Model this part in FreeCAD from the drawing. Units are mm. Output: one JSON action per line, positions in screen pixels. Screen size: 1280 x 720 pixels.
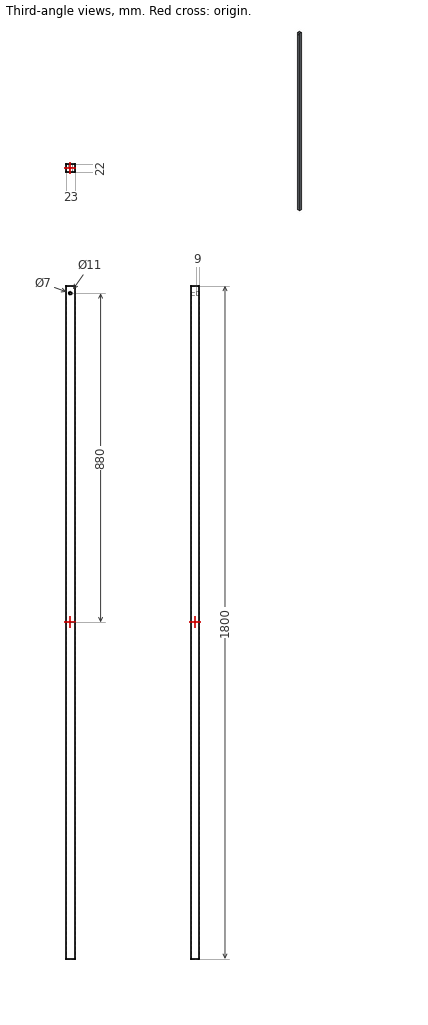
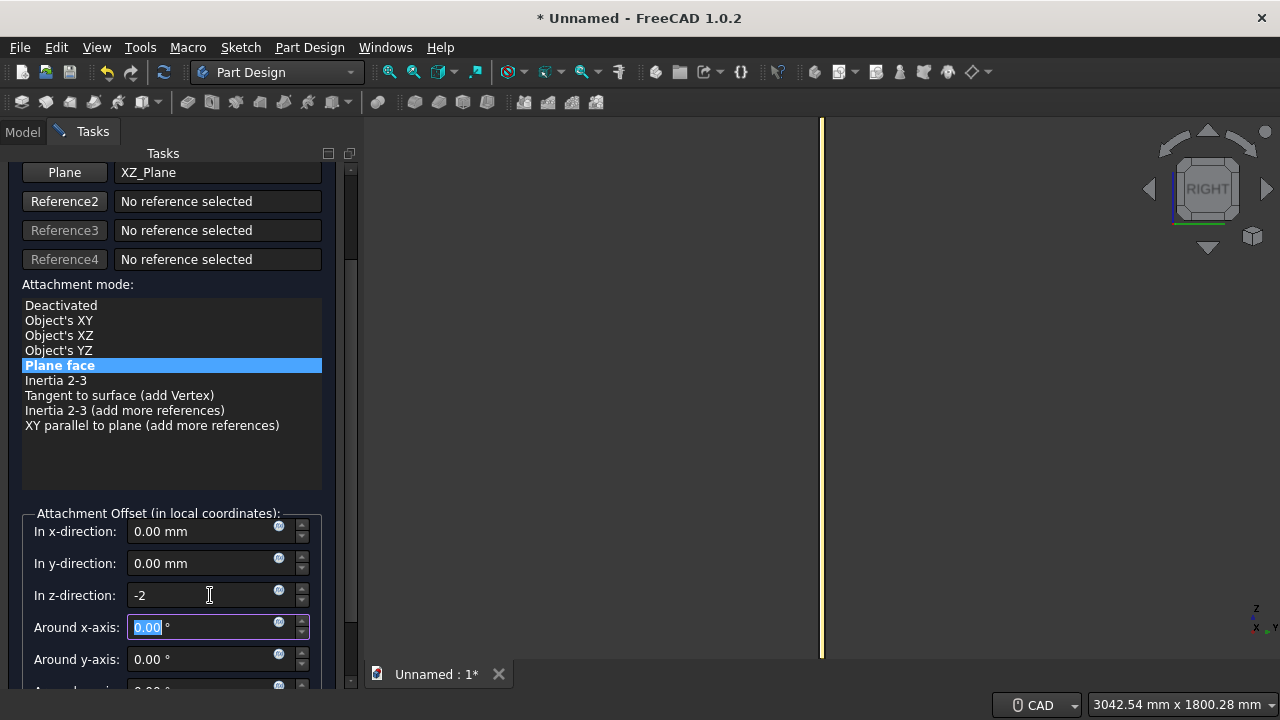
{"action": "scroll", "coordinate": [351, 426], "scroll_direction": "up", "scroll_amount": 3}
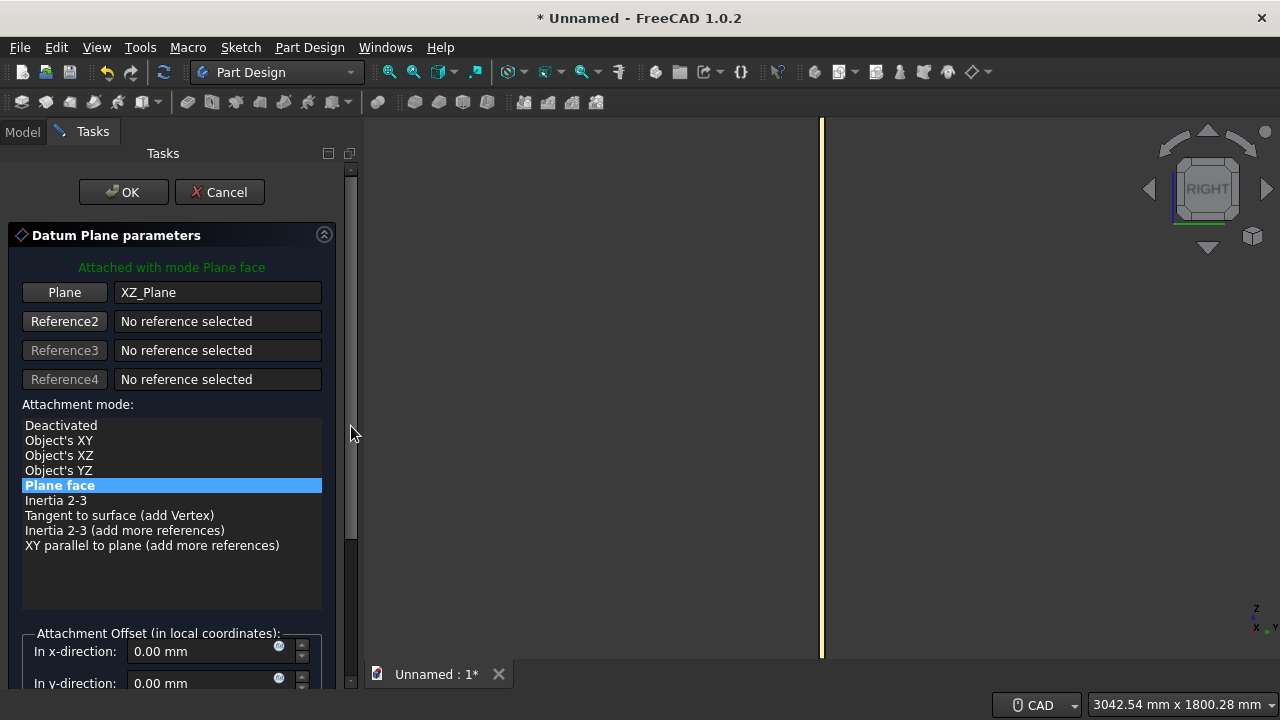
{"action": "left_click", "coordinate": [124, 192]}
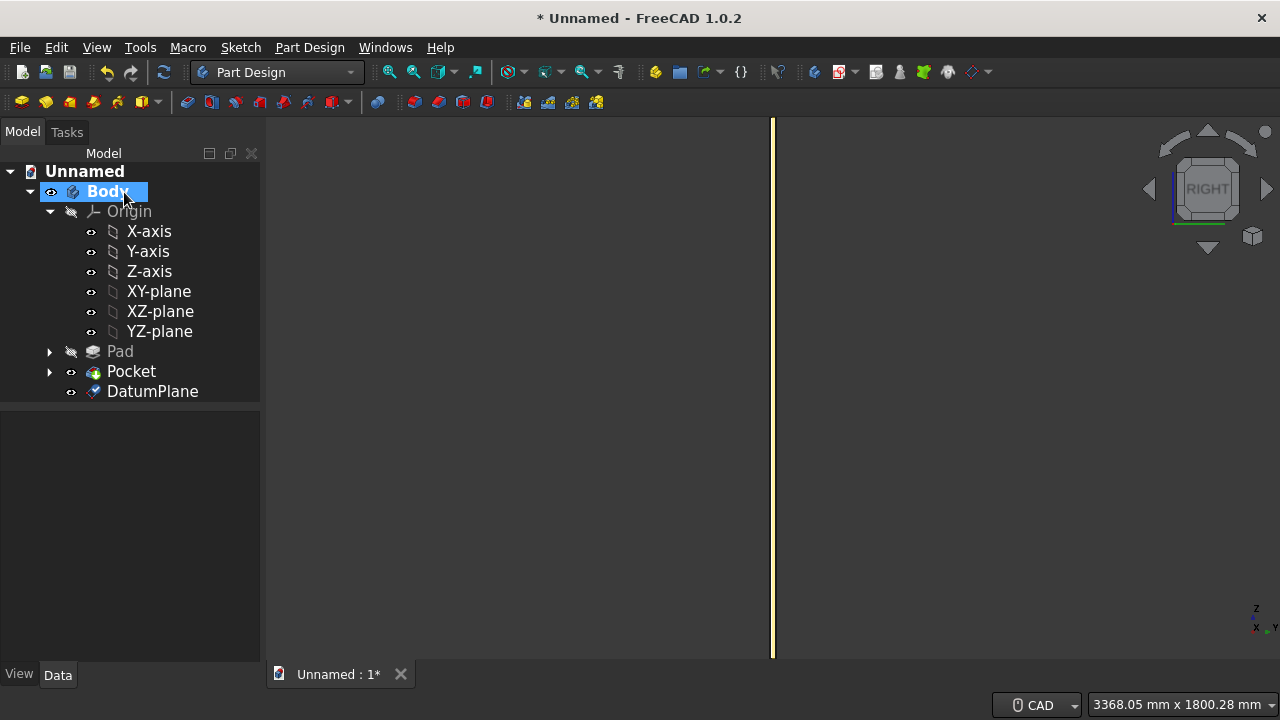
{"action": "left_click", "coordinate": [116, 392]}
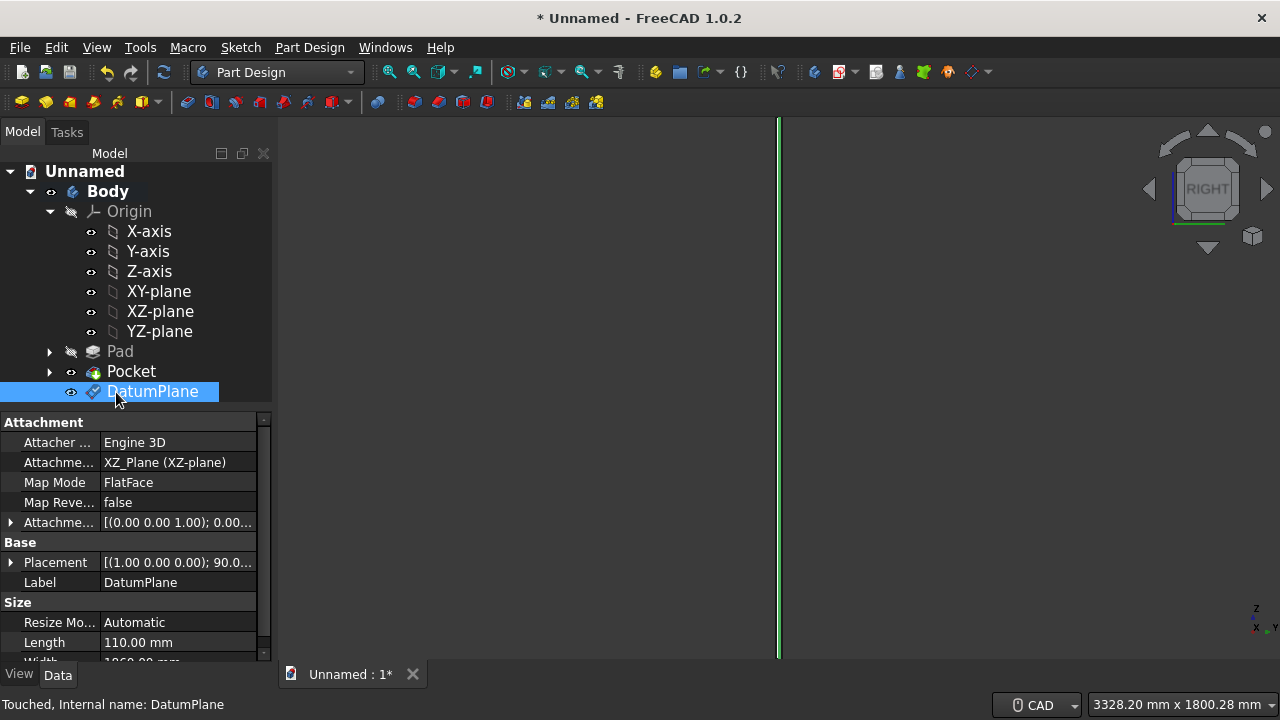
{"action": "left_click", "coordinate": [840, 72]}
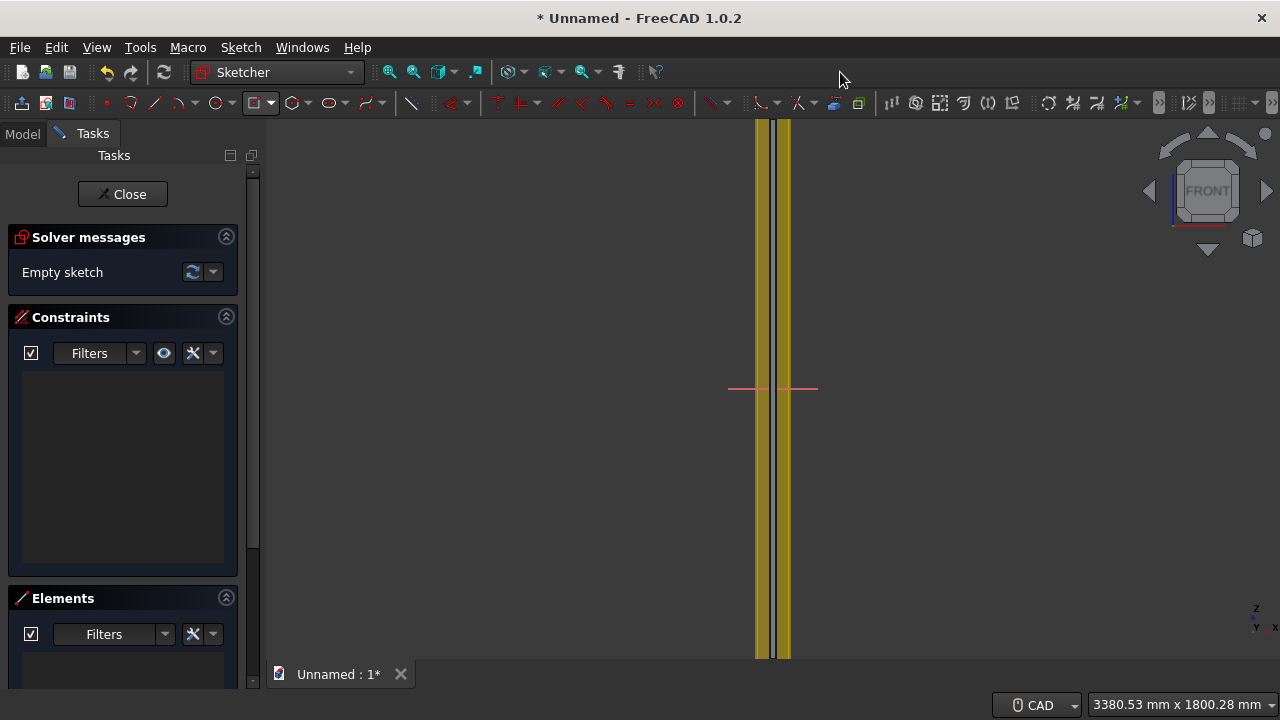
{"action": "left_click", "coordinate": [70, 104]}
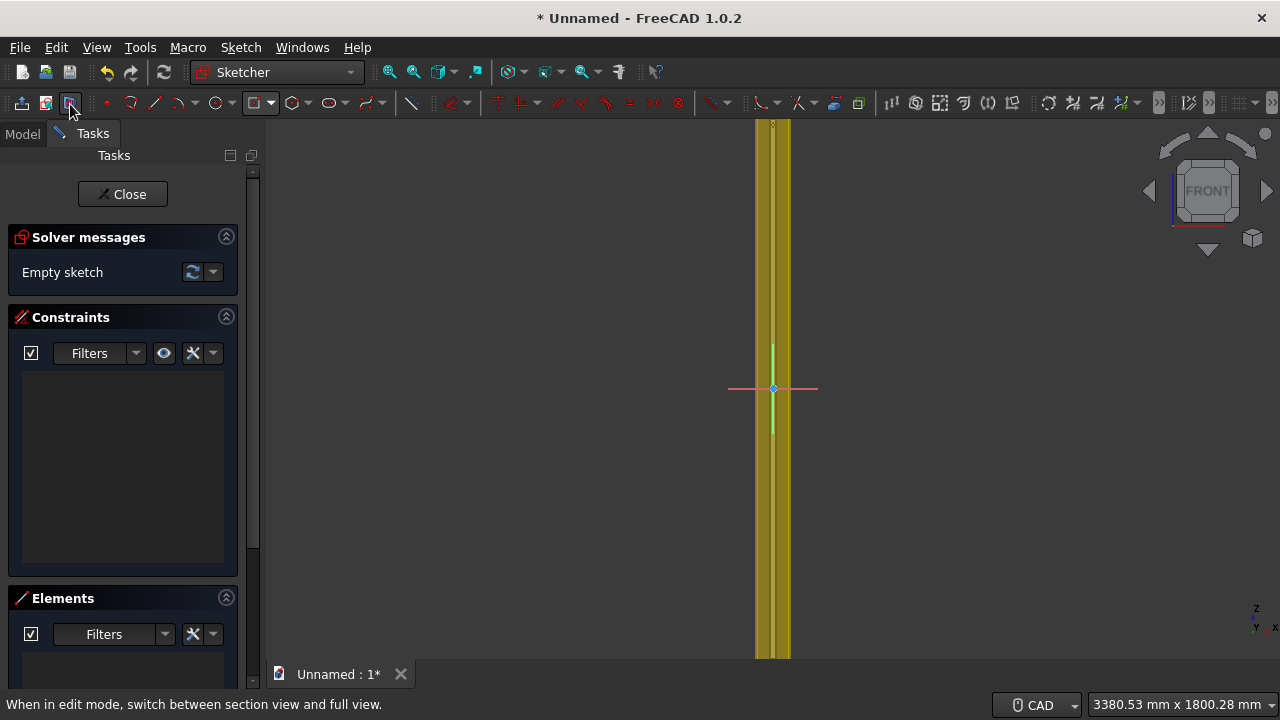
{"action": "scroll", "coordinate": [704, 389], "scroll_direction": "down", "scroll_amount": 5}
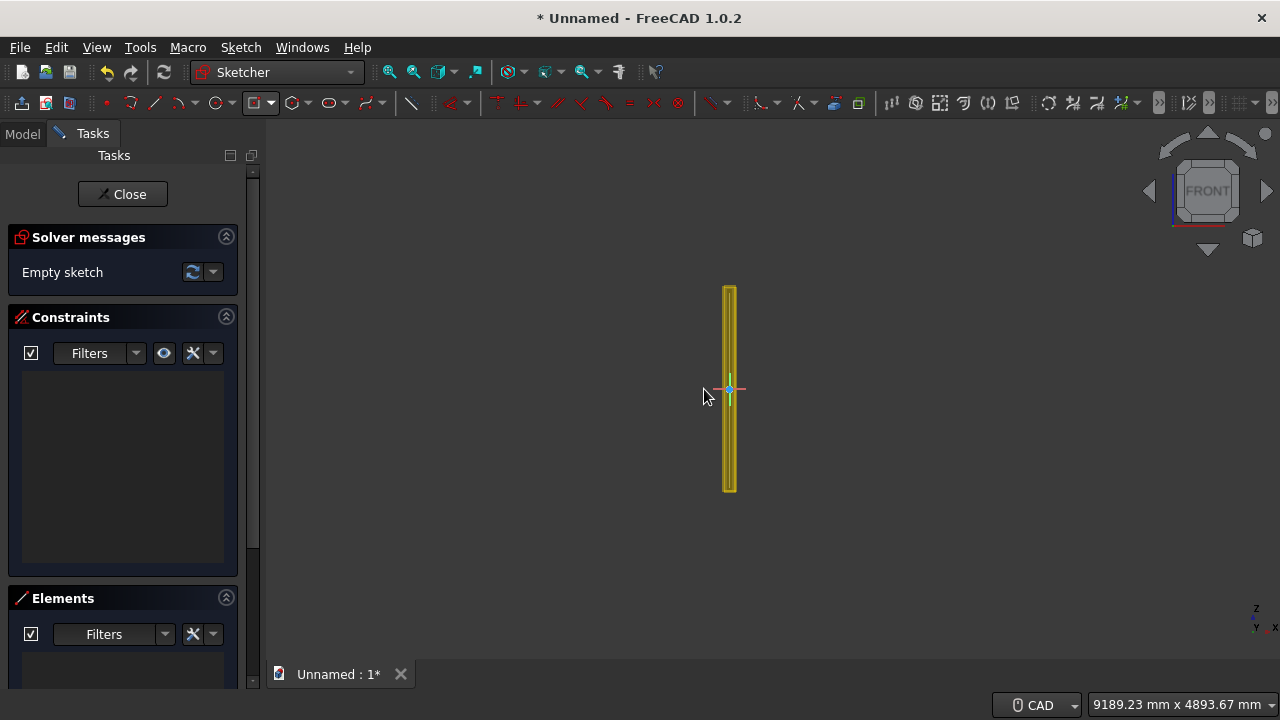
{"action": "scroll", "coordinate": [731, 287], "scroll_direction": "up", "scroll_amount": 15}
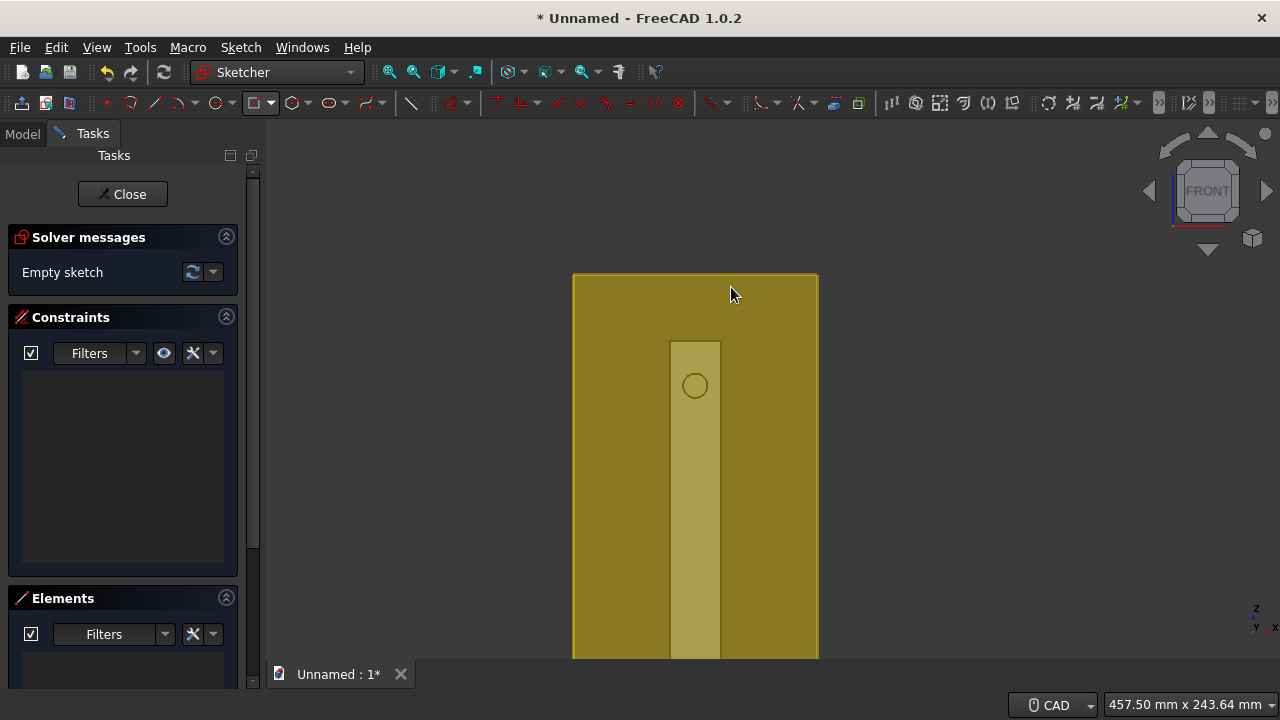
{"action": "scroll", "coordinate": [695, 386], "scroll_direction": "up", "scroll_amount": 15}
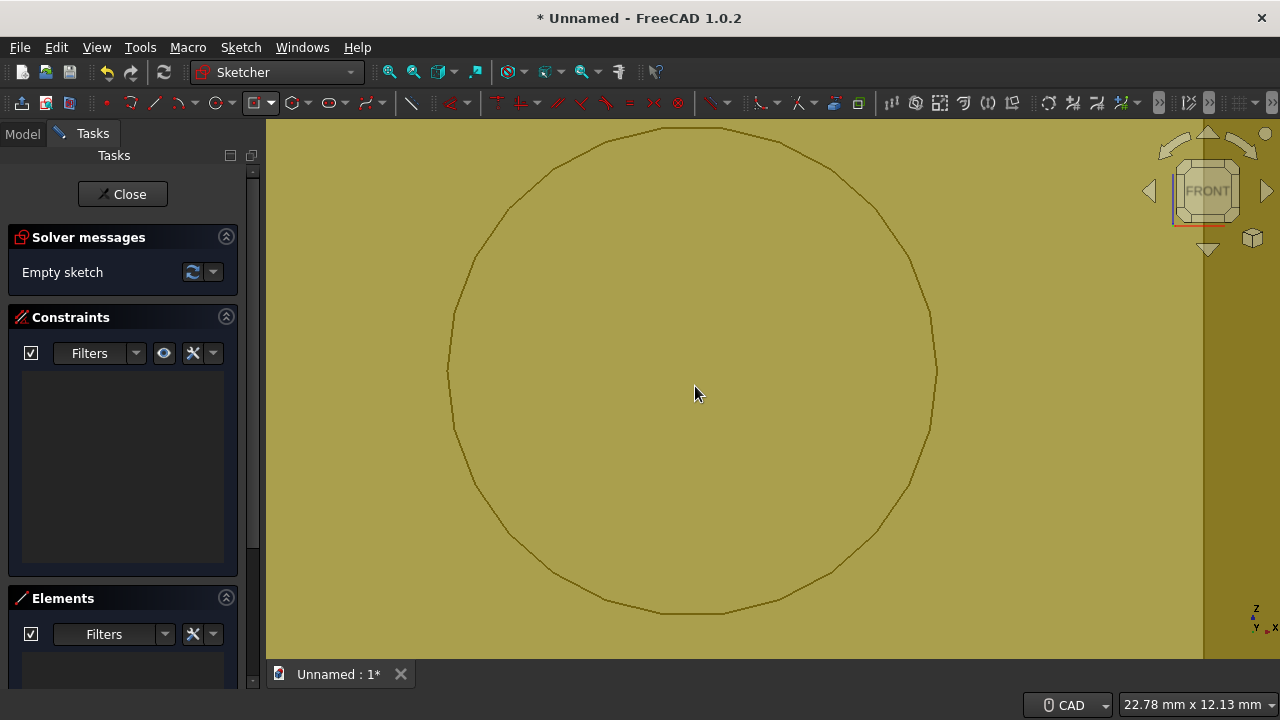
{"action": "left_click", "coordinate": [216, 104]}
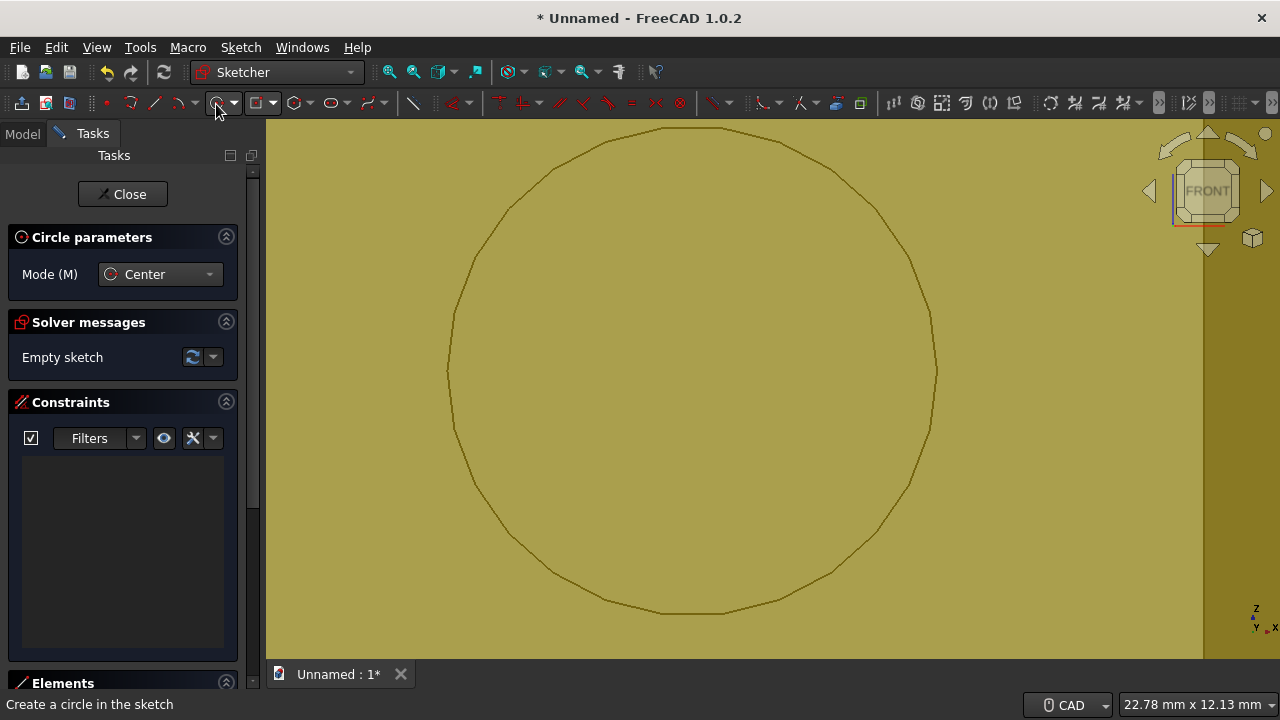
{"action": "left_click", "coordinate": [692, 371]}
{"action": "left_click", "coordinate": [802, 261]}
{"action": "key", "text": "Escape"}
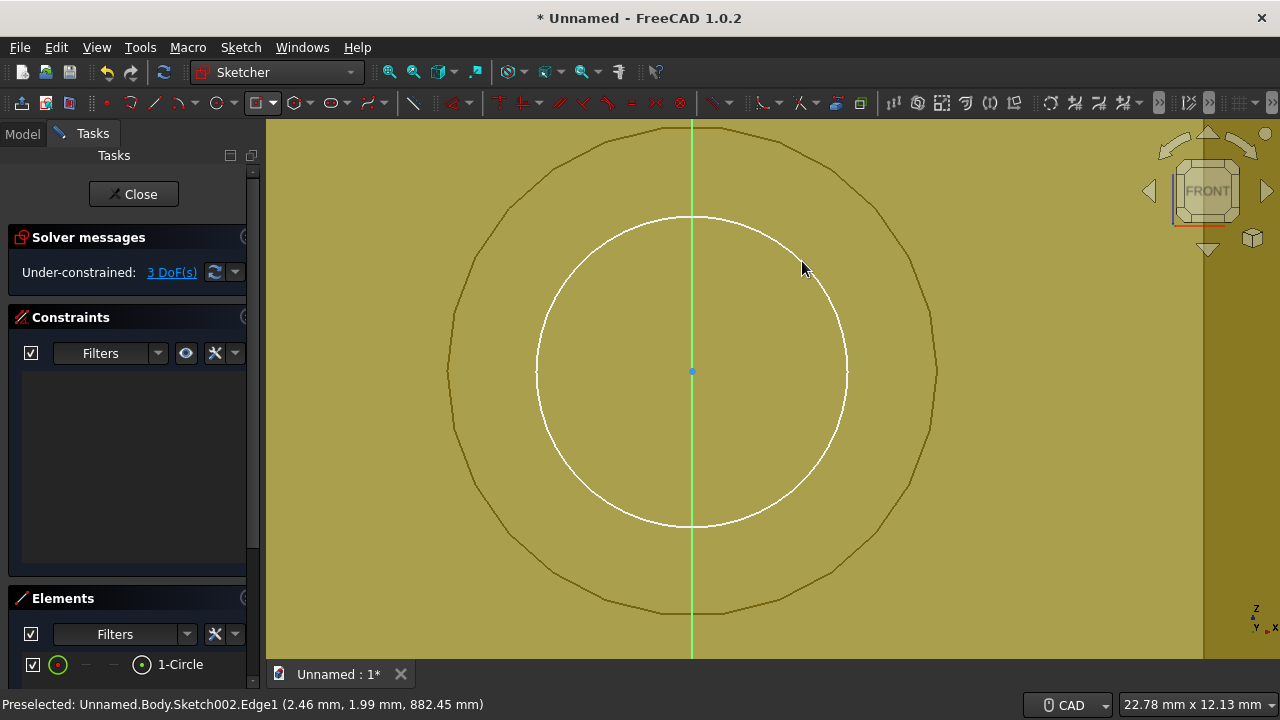
{"action": "left_click", "coordinate": [692, 372]}